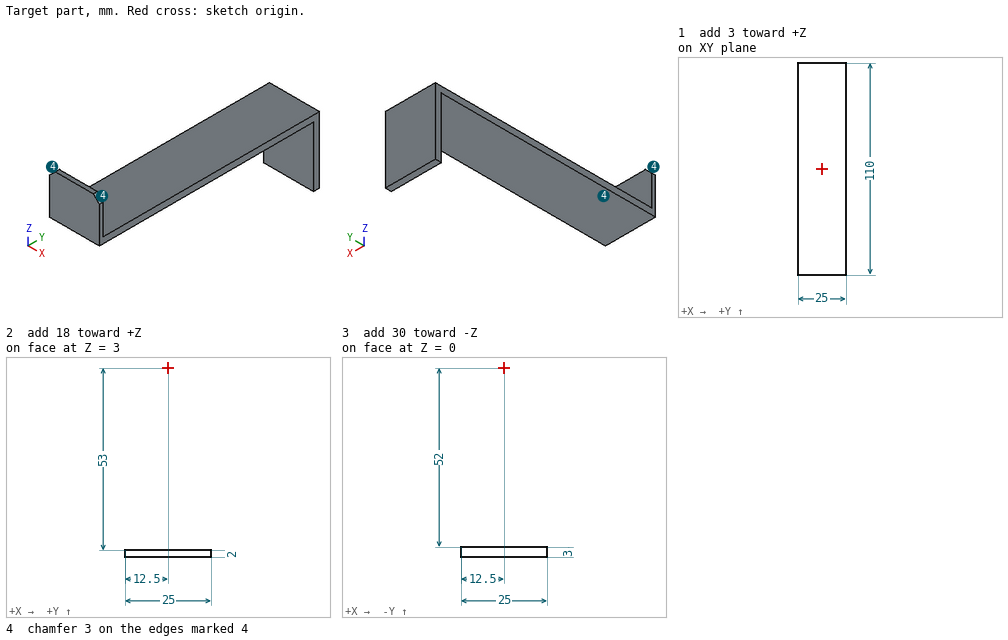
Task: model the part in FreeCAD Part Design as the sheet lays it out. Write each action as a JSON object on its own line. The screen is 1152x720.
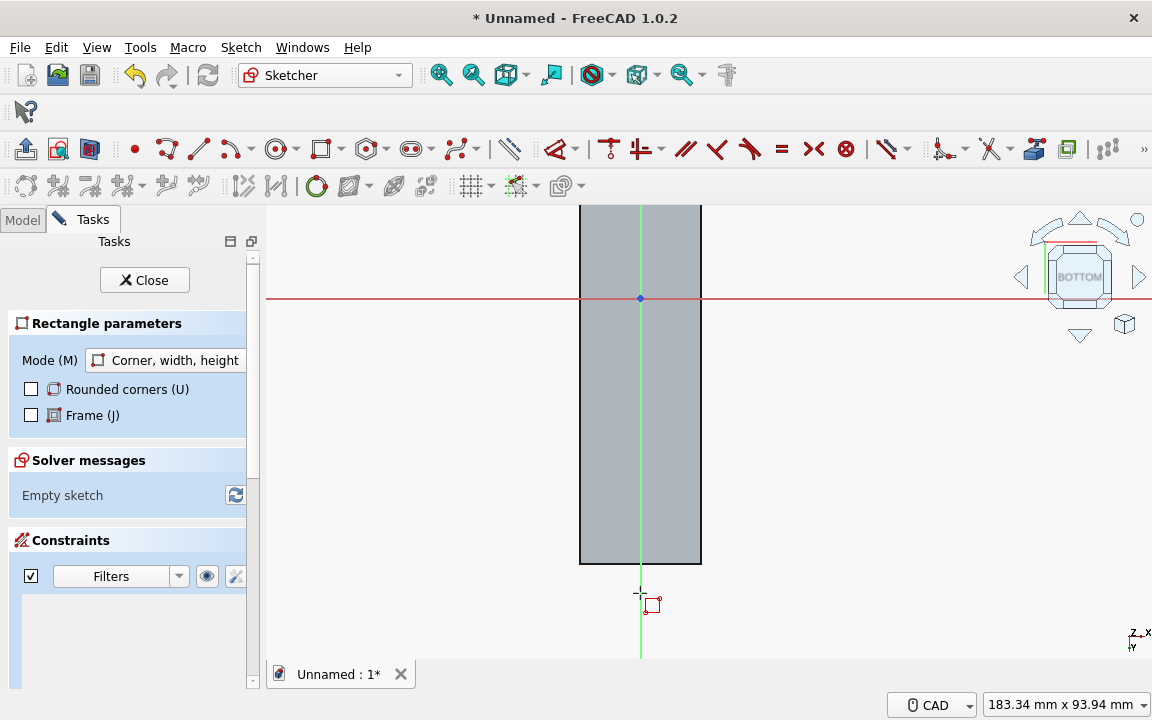
{"action": "left_click", "coordinate": [580, 550]}
{"action": "mouse_move", "coordinate": [701, 564]}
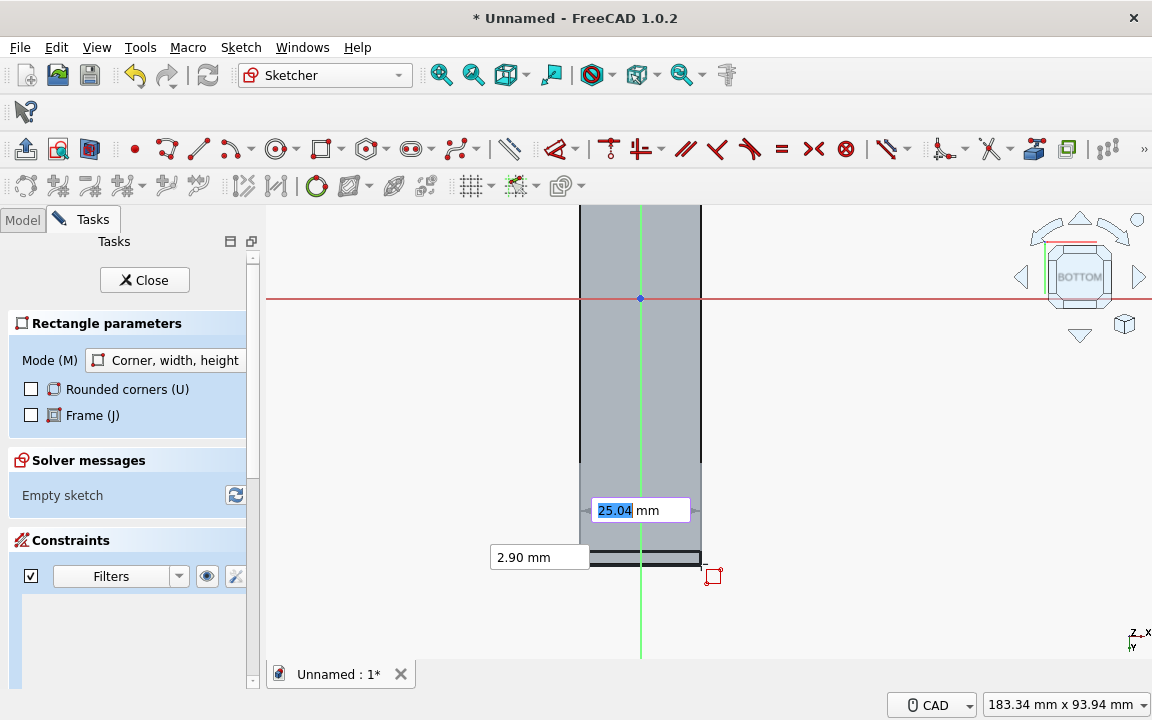
{"action": "type", "text": "25"}
{"action": "key", "text": "Tab"}
{"action": "type", "text": "3"}
{"action": "key", "text": "Return"}
{"action": "key", "text": "Escape"}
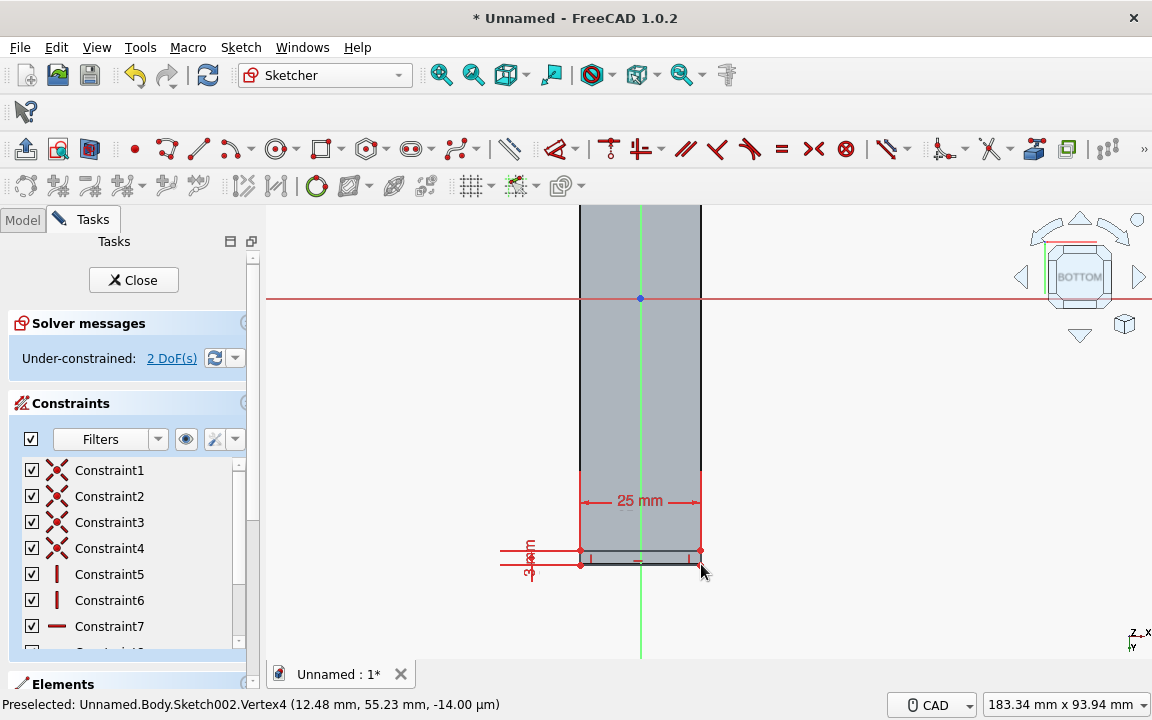
{"action": "key", "text": "d"}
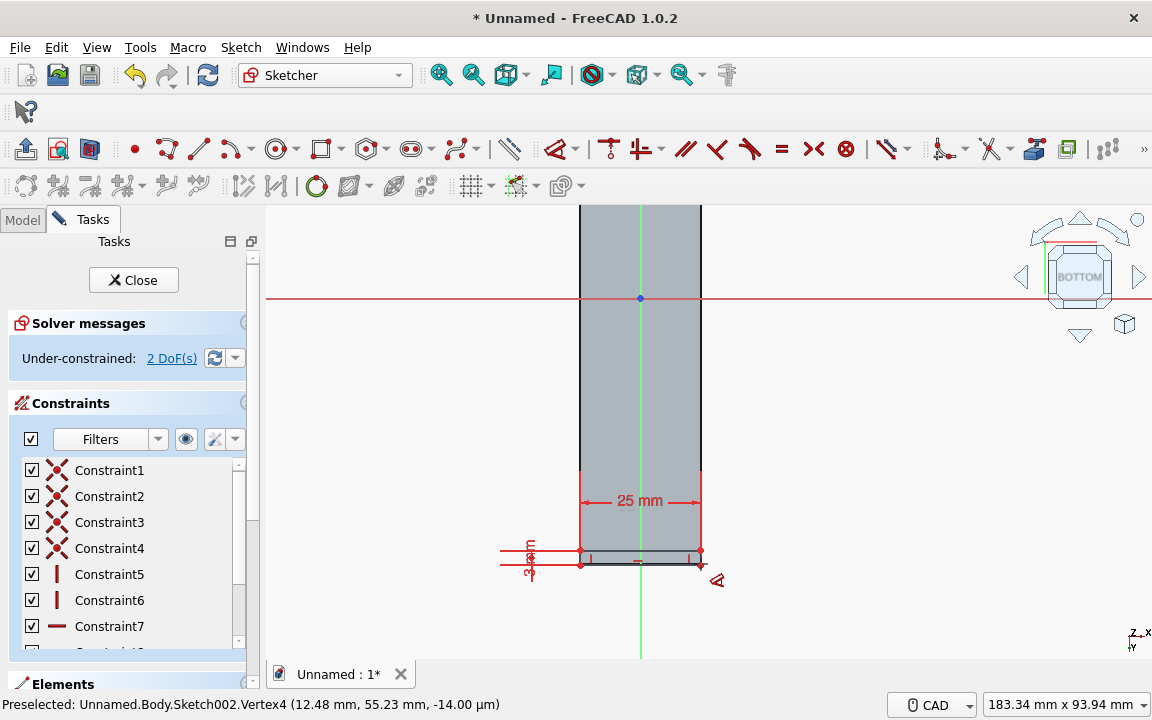
{"action": "left_click", "coordinate": [580, 551]}
{"action": "left_click", "coordinate": [546, 425]}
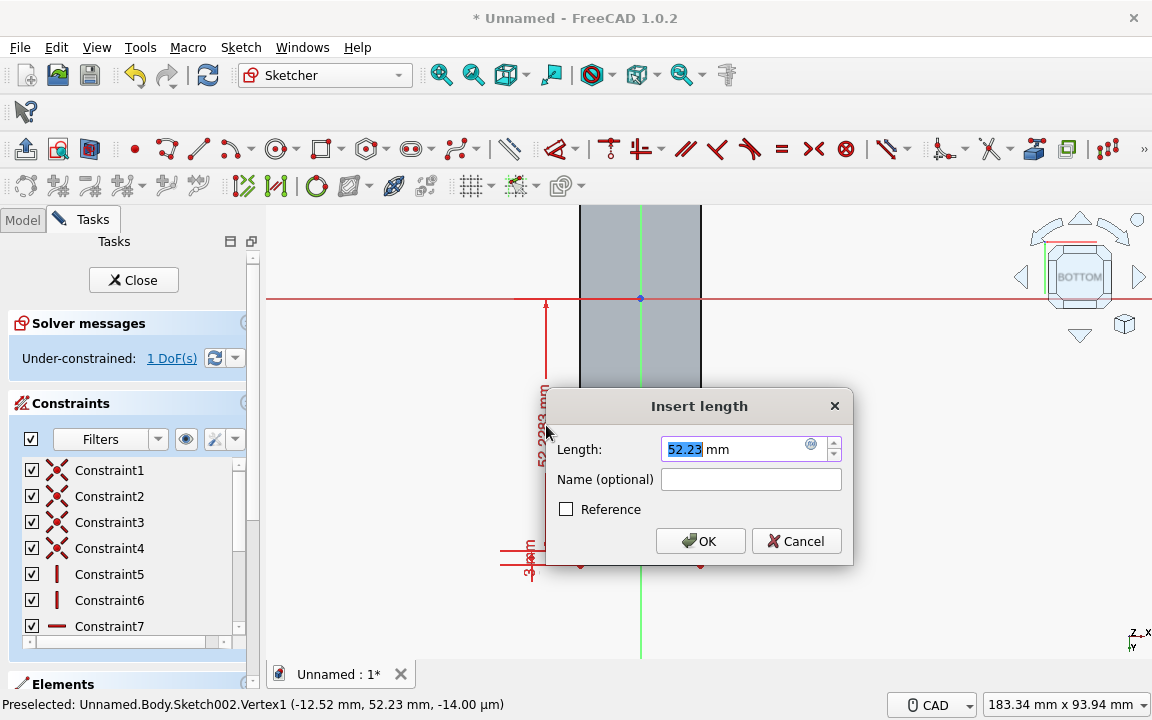
{"action": "type", "text": "52"}
{"action": "key", "text": "Return"}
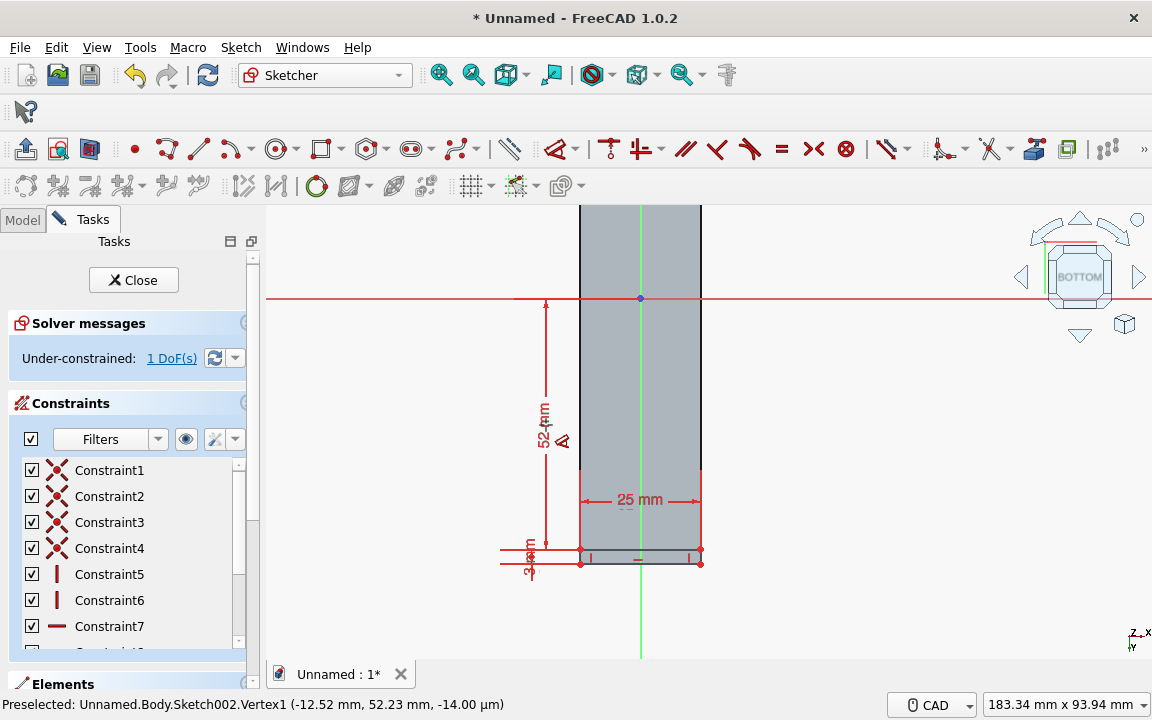
{"action": "left_click", "coordinate": [580, 550]}
{"action": "left_click", "coordinate": [610, 265]}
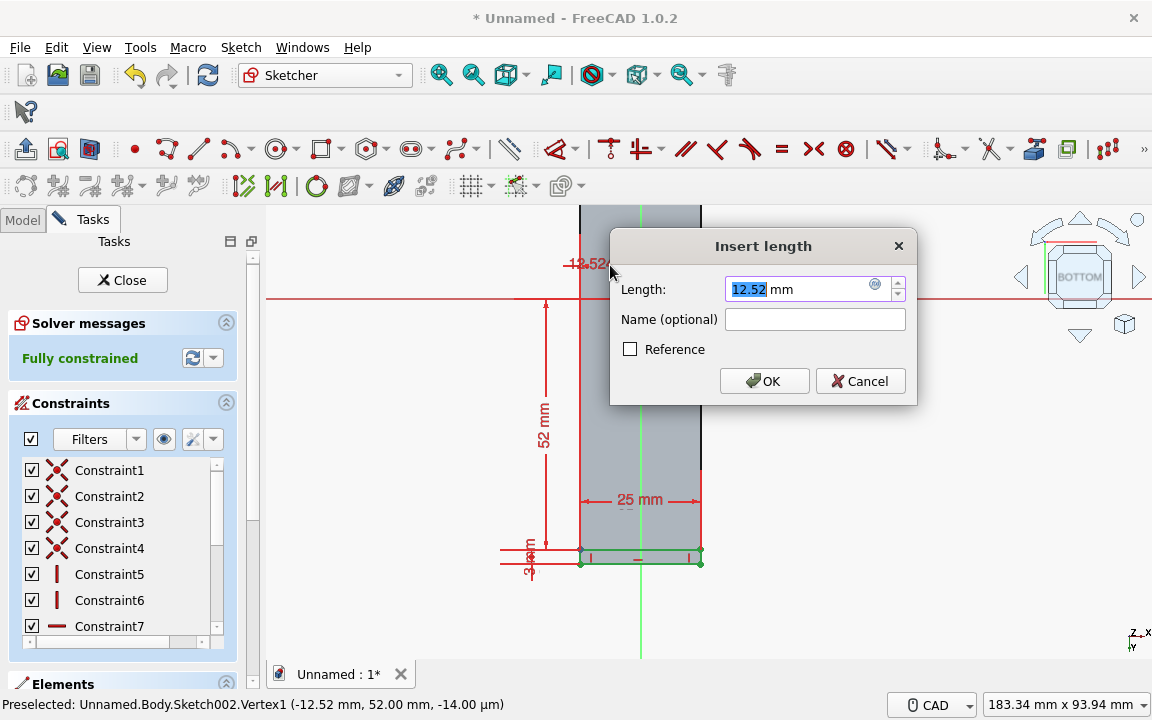
{"action": "type", "text": "12.5"}
{"action": "key", "text": "Return"}
{"action": "key", "text": "Escape"}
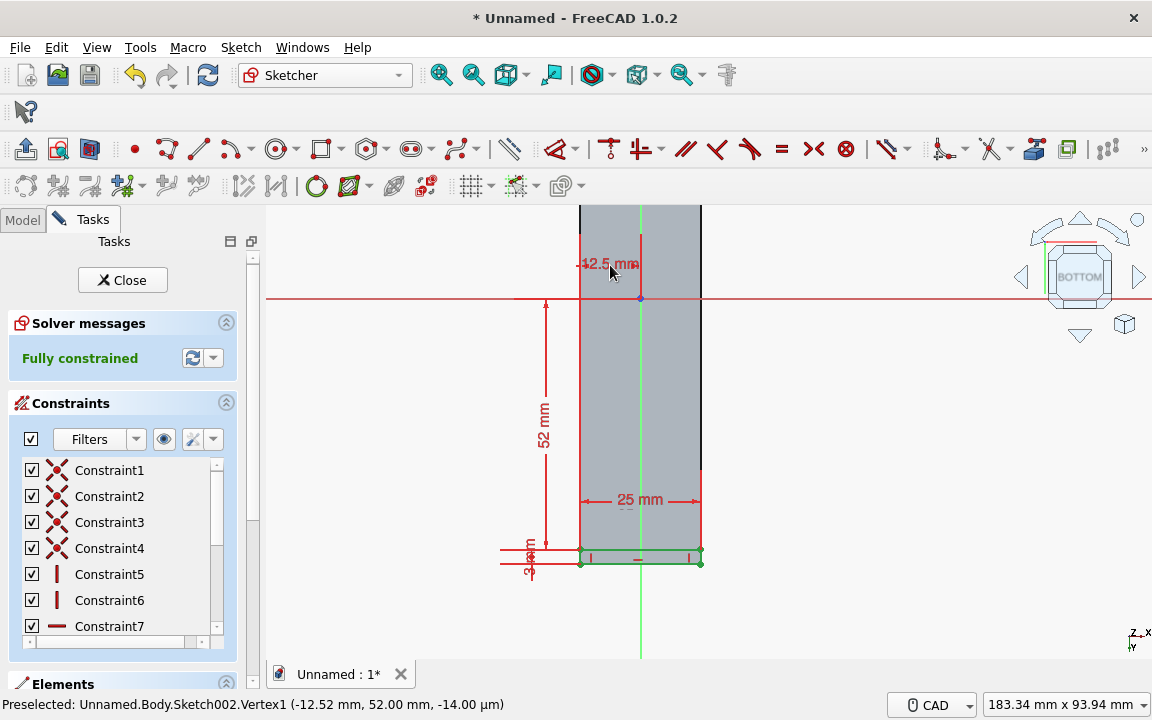
{"action": "left_click", "coordinate": [123, 280]}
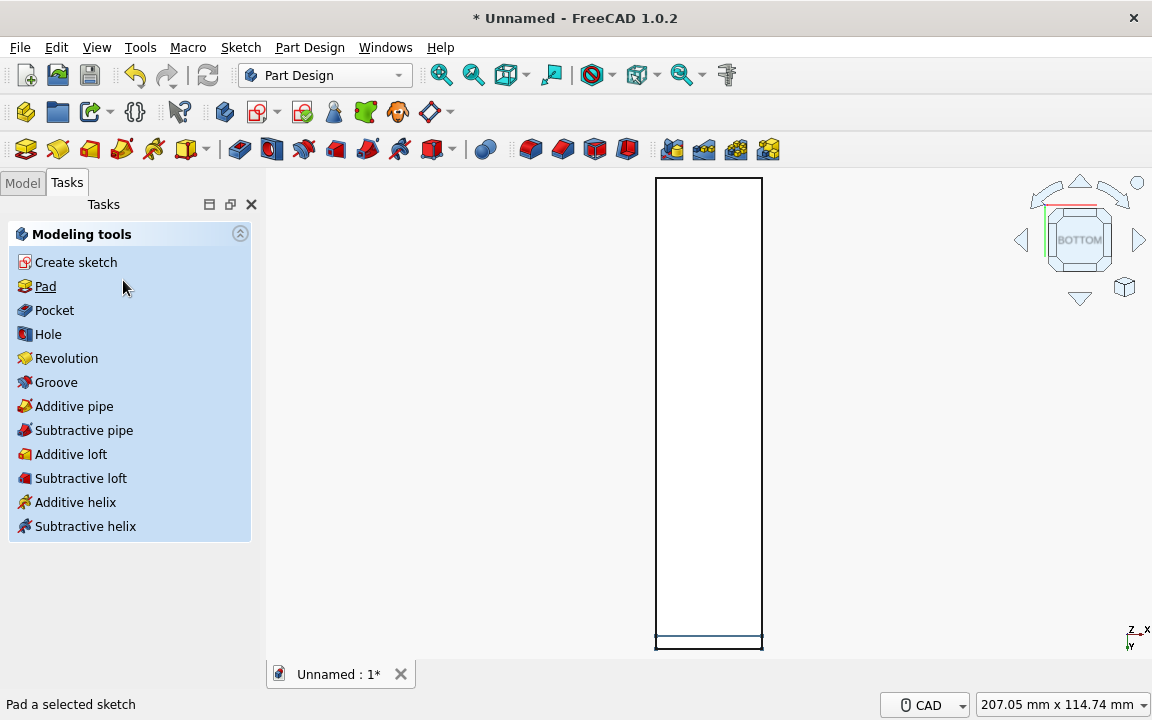
{"action": "left_click", "coordinate": [26, 150]}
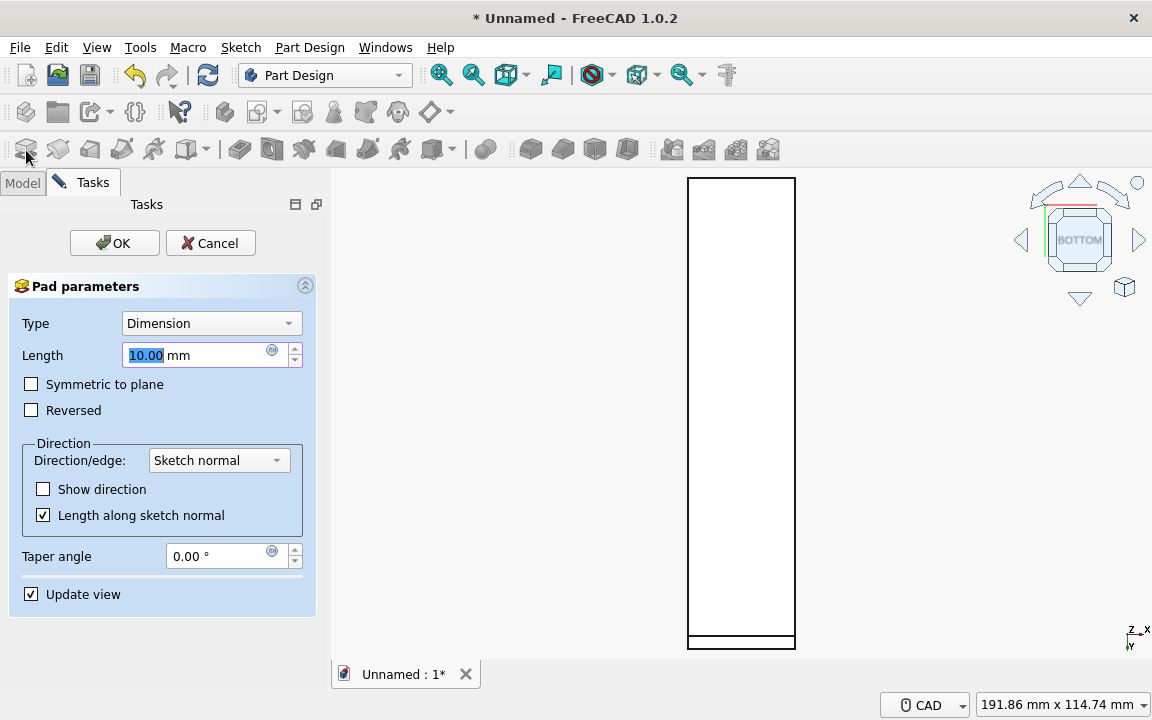
{"action": "type", "text": "30"}
{"action": "key", "text": "Tab"}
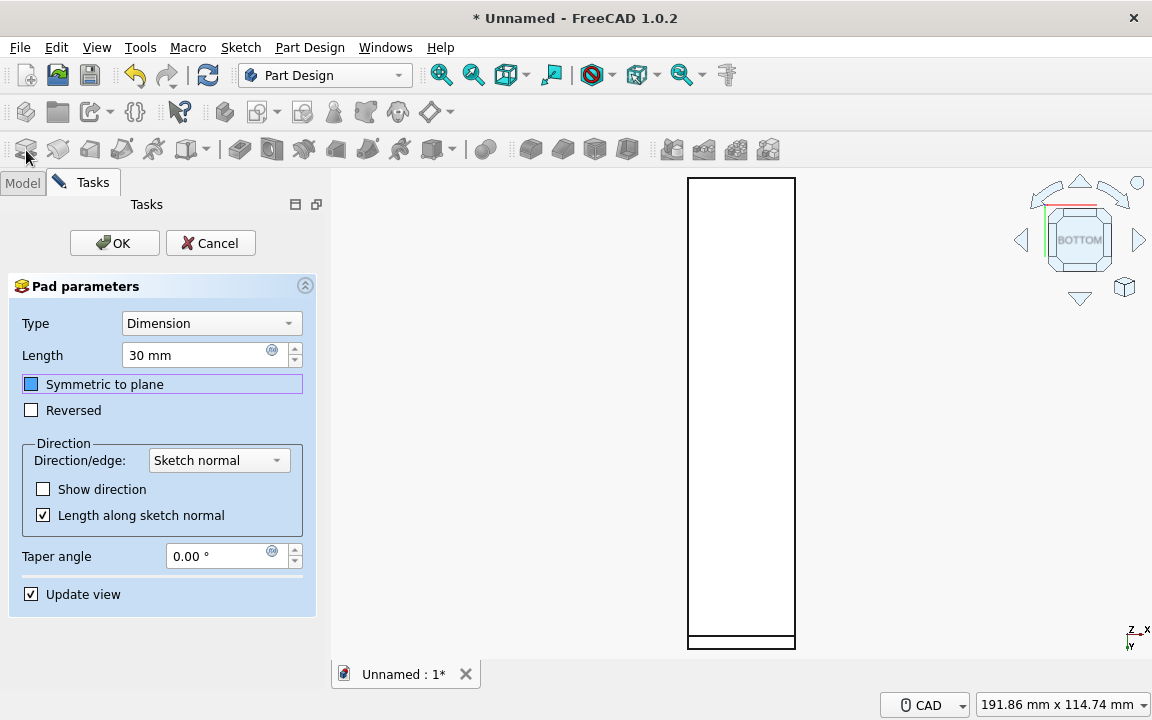
{"action": "left_click", "coordinate": [115, 243]}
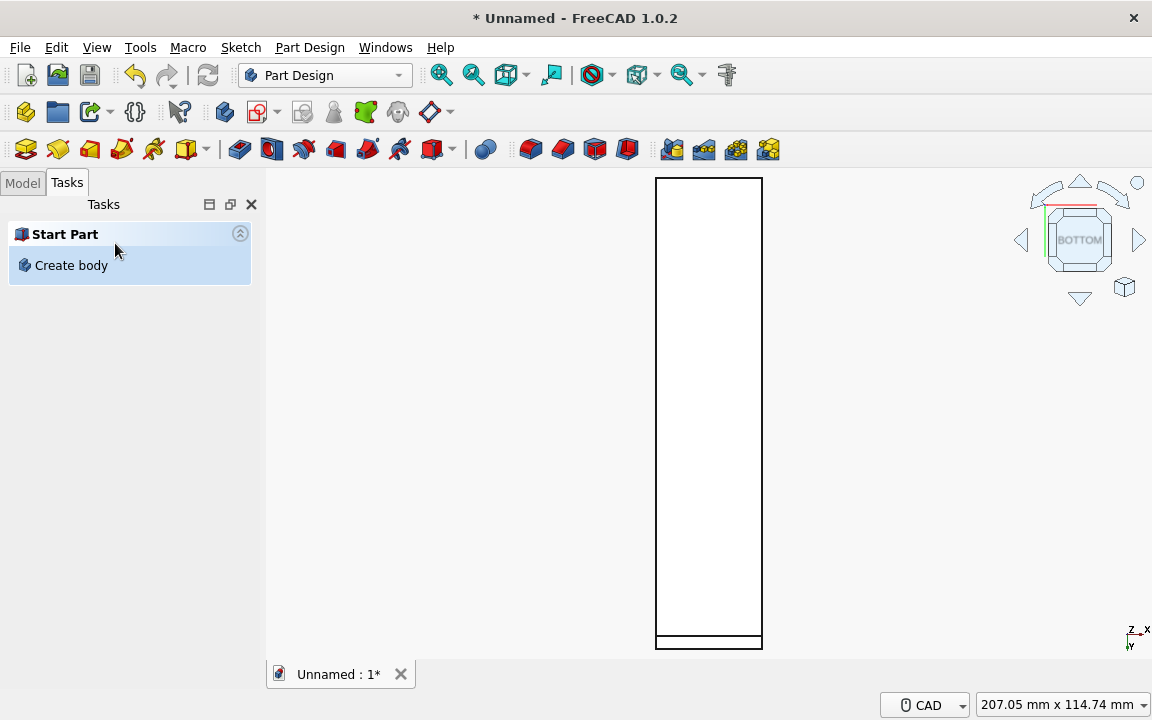
{"action": "key", "text": "0"}